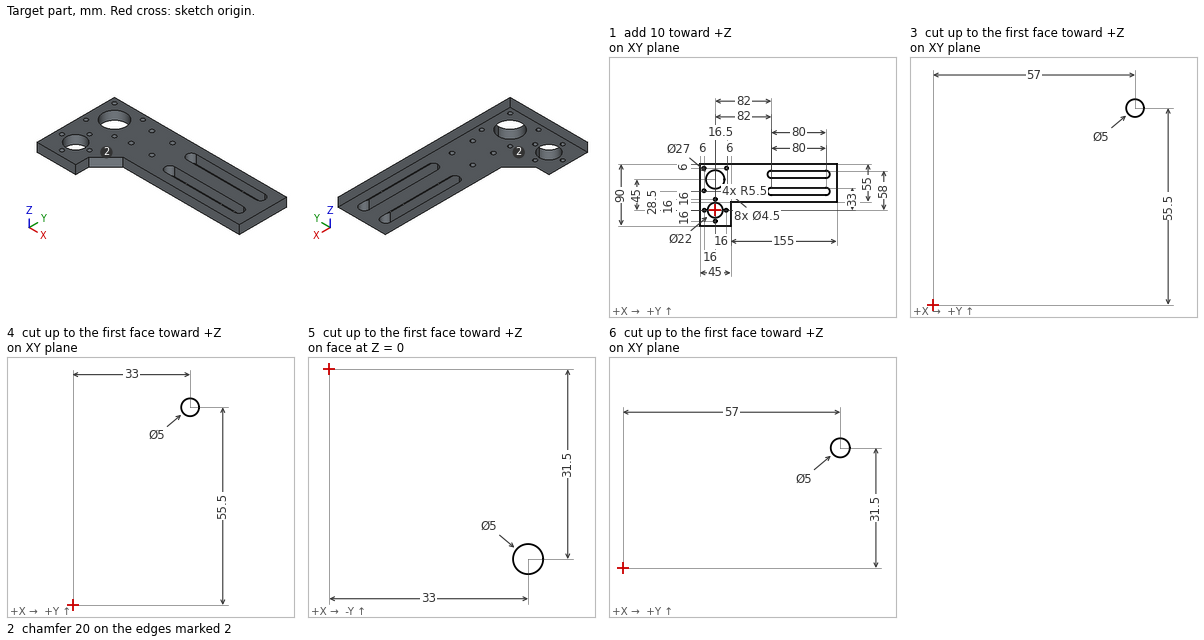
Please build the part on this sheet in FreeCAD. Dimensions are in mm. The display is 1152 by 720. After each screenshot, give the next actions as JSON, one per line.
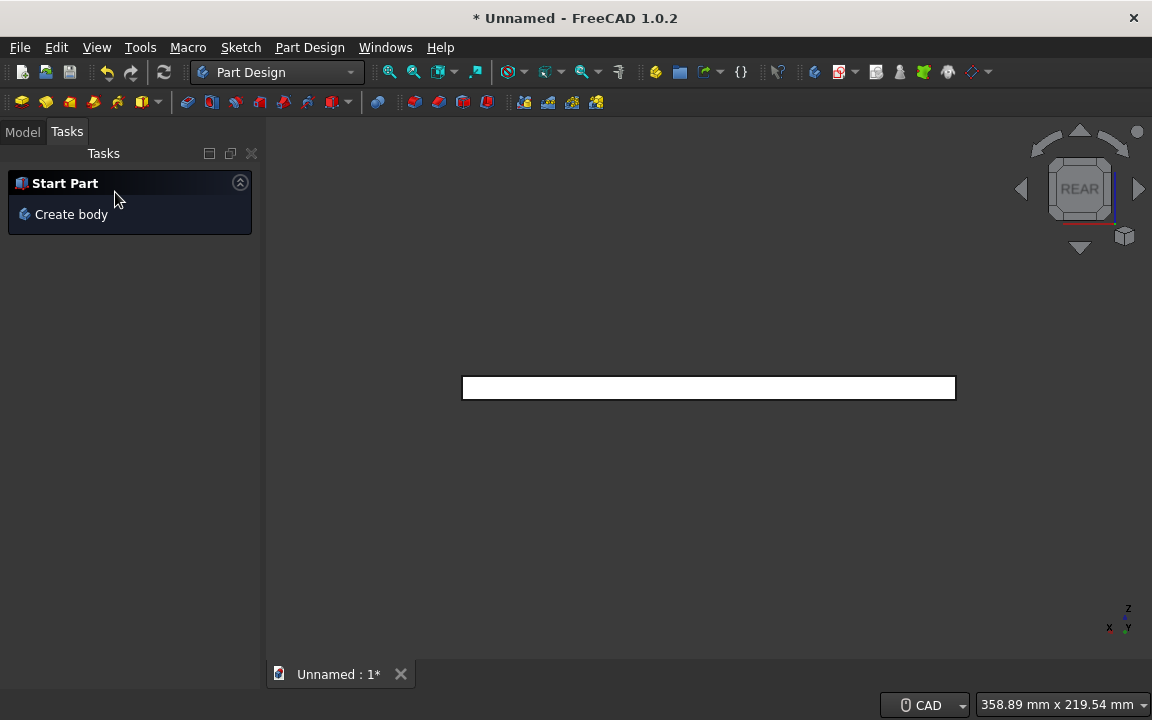
{"action": "key", "text": "6"}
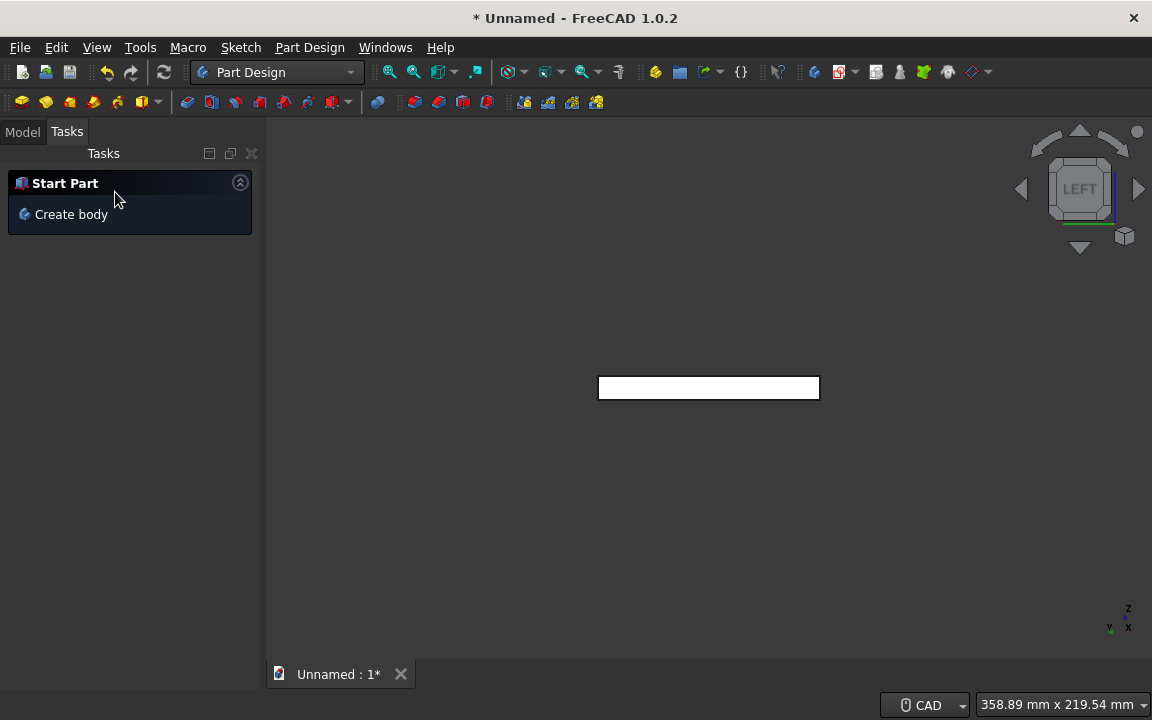
{"action": "key", "text": "v f"}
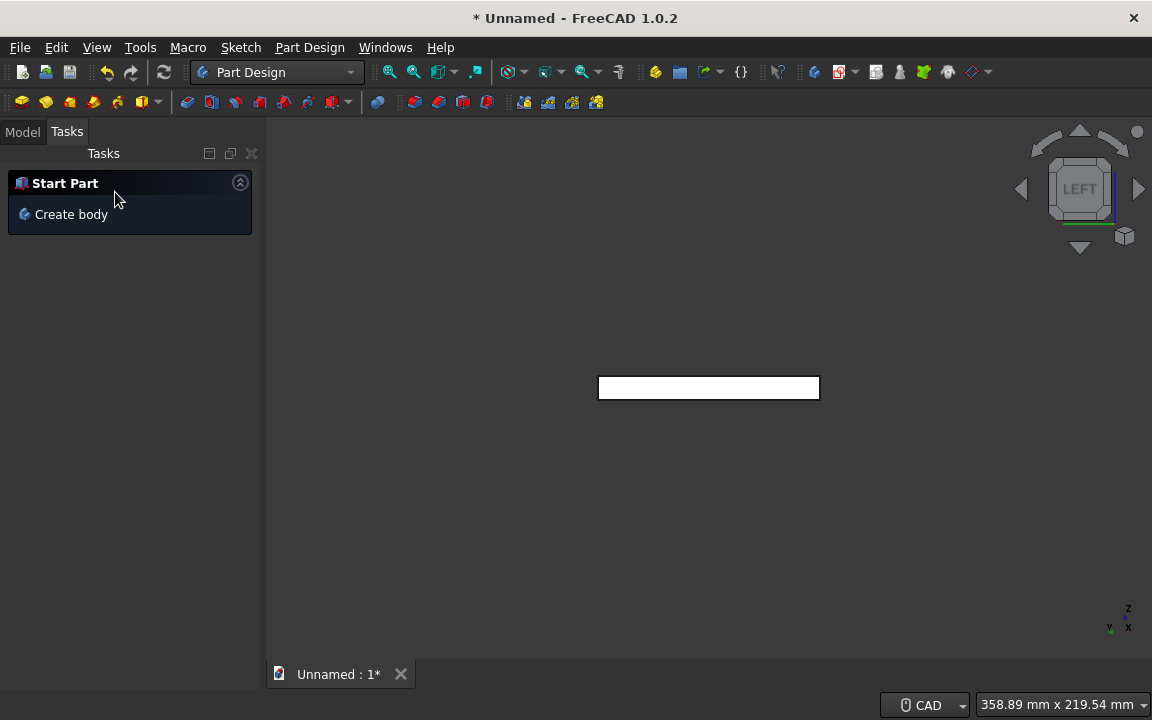
{"action": "key", "text": "v 3"}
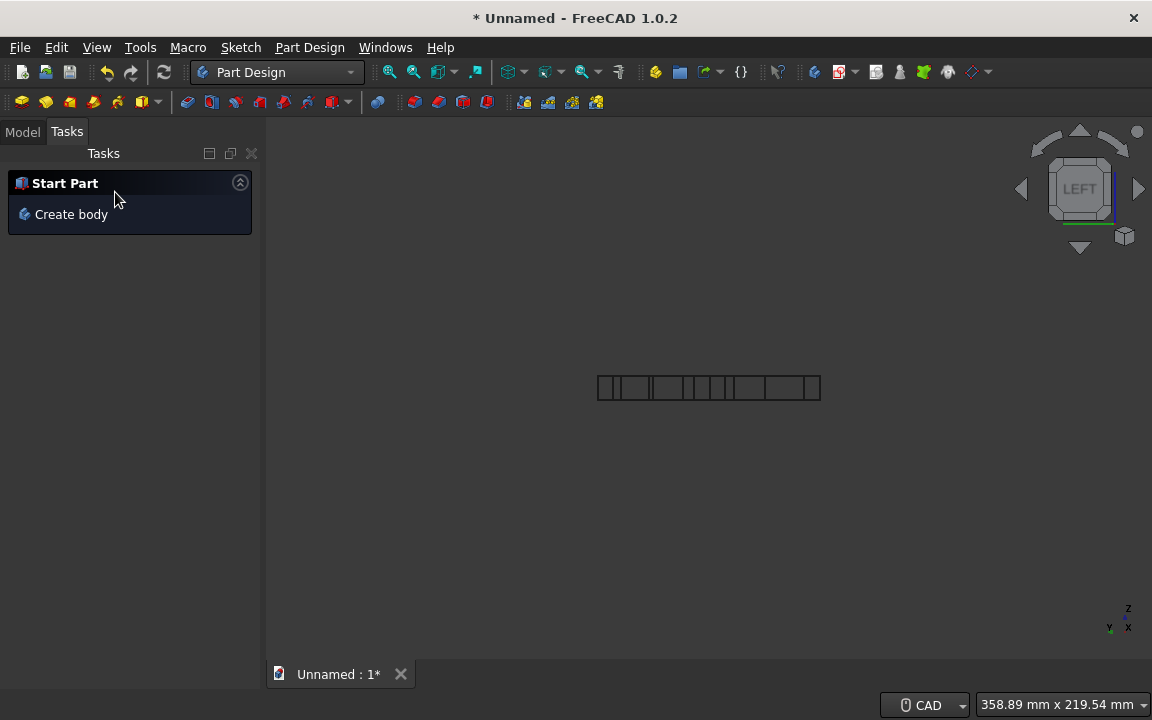
{"action": "key", "text": "0"}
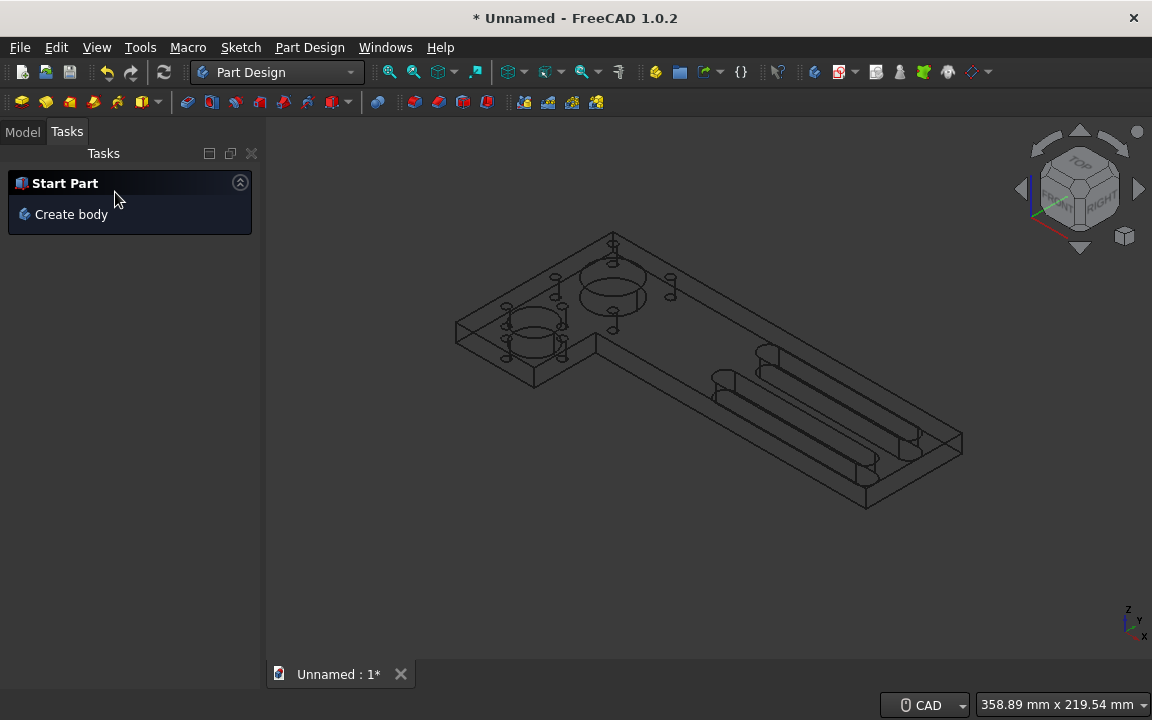
{"action": "left_click", "coordinate": [596, 342]}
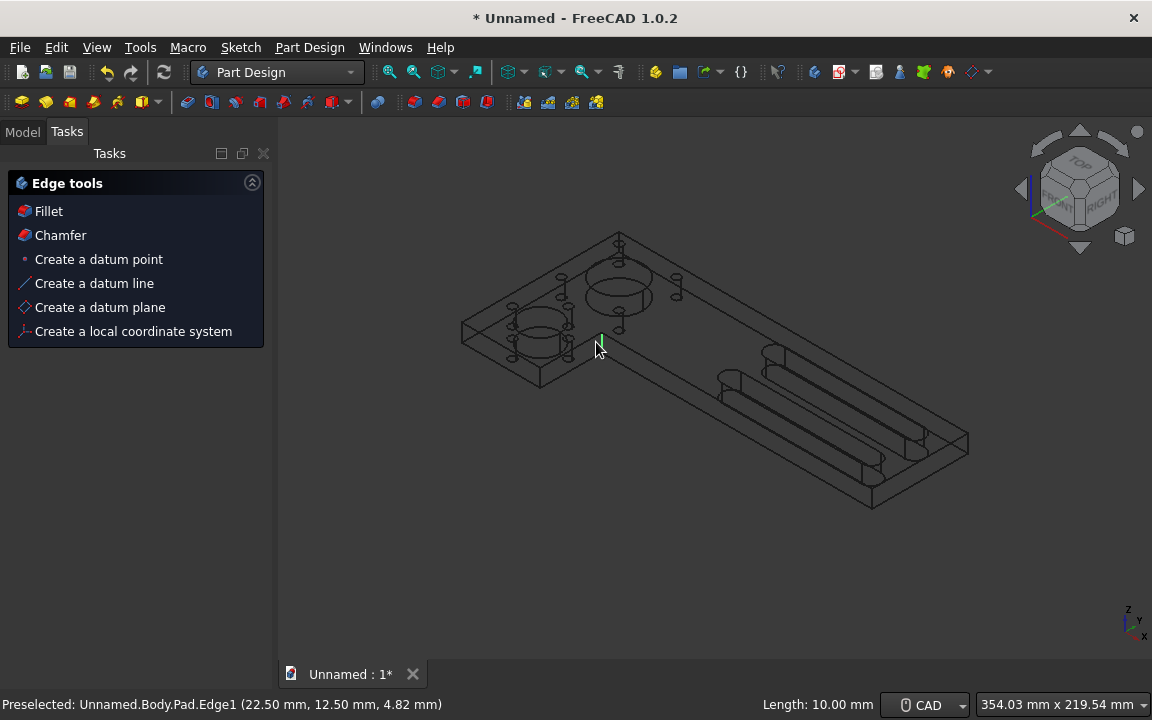
{"action": "key", "text": "v 1"}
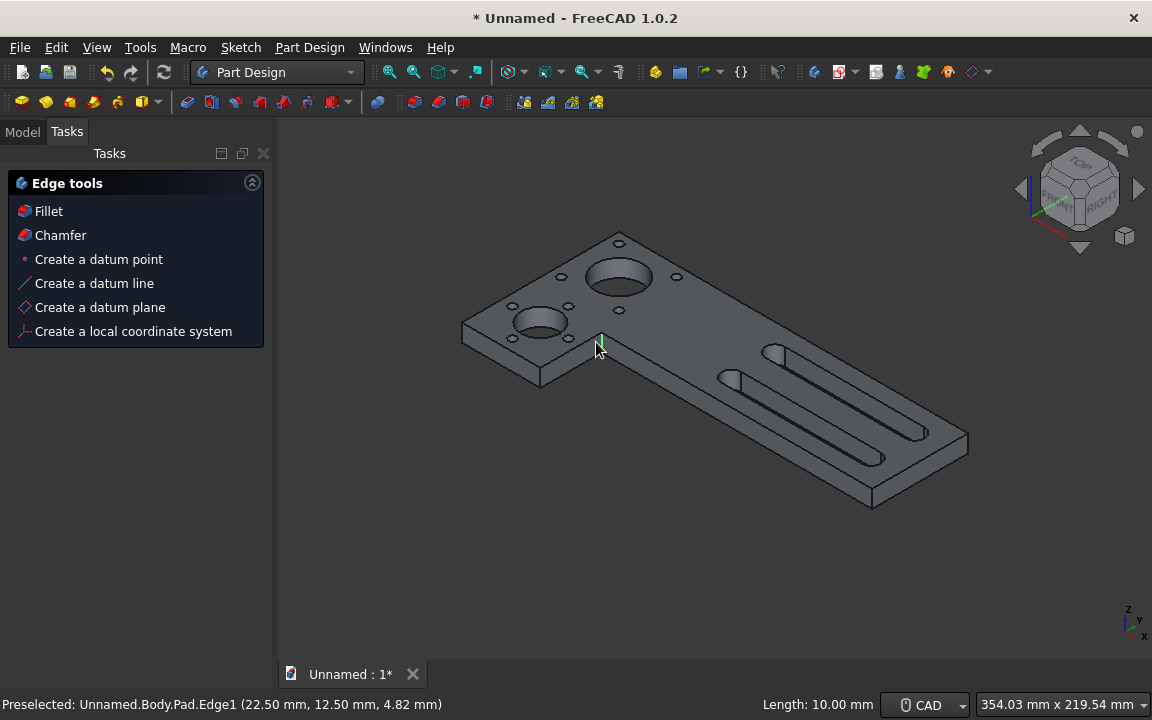
{"action": "left_click", "coordinate": [440, 102]}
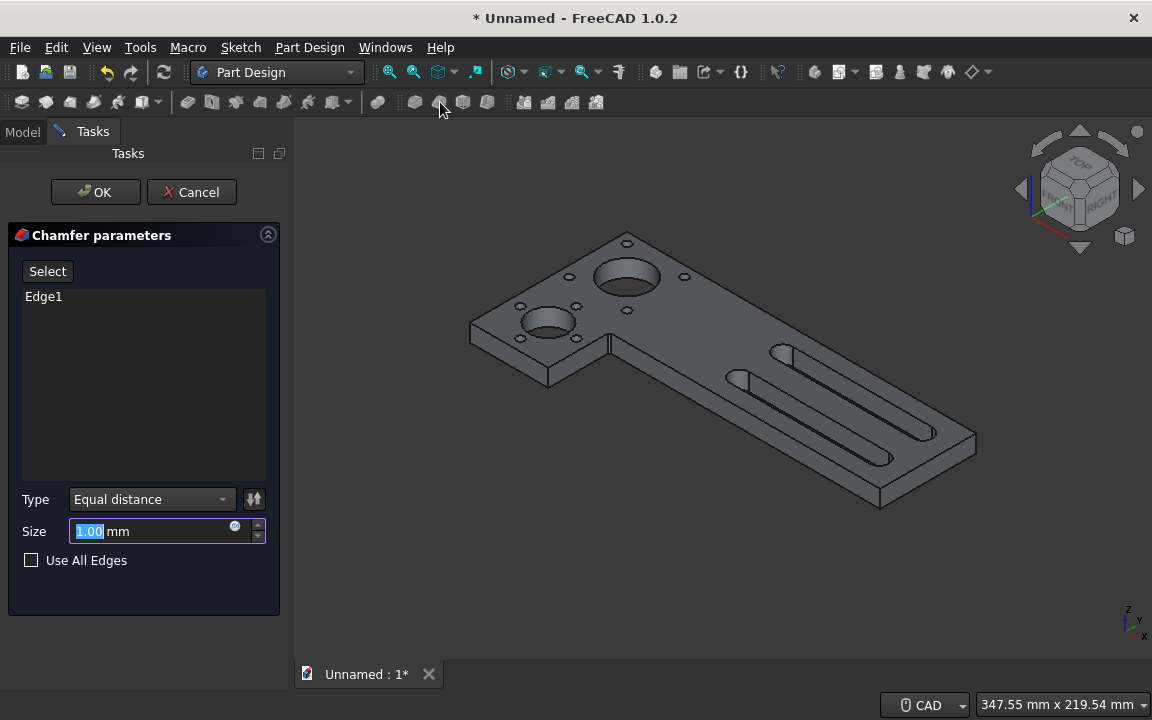
{"action": "type", "text": "20"}
{"action": "key", "text": "Tab"}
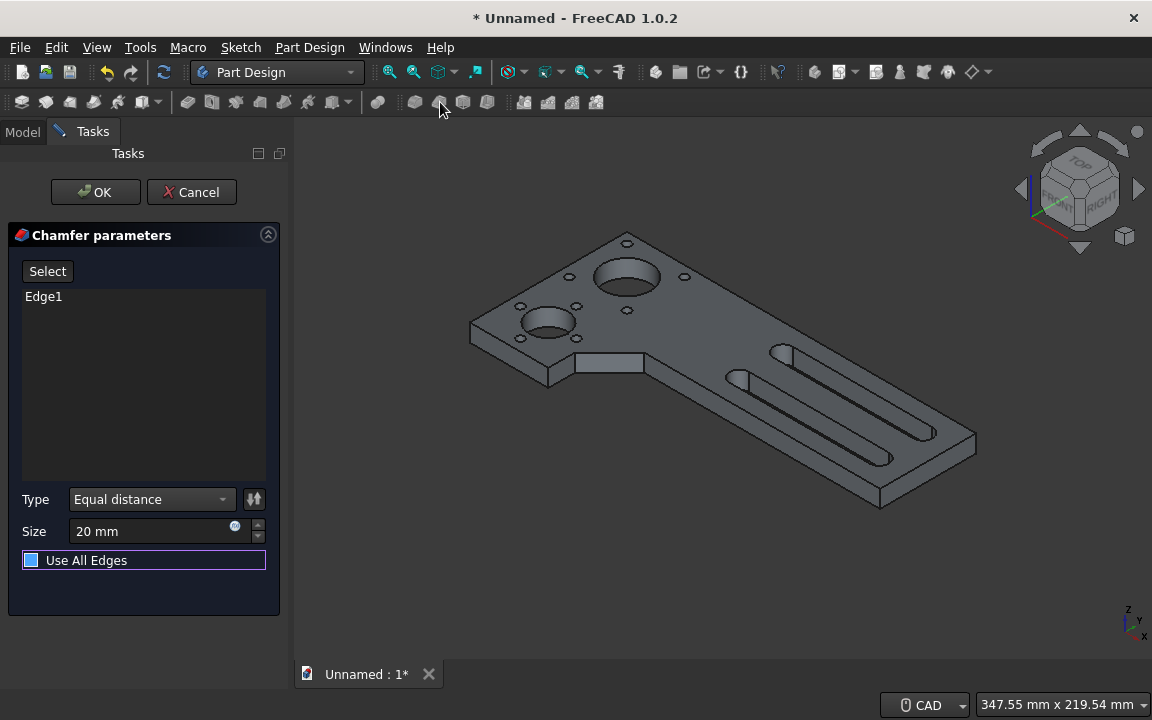
{"action": "left_click", "coordinate": [96, 192]}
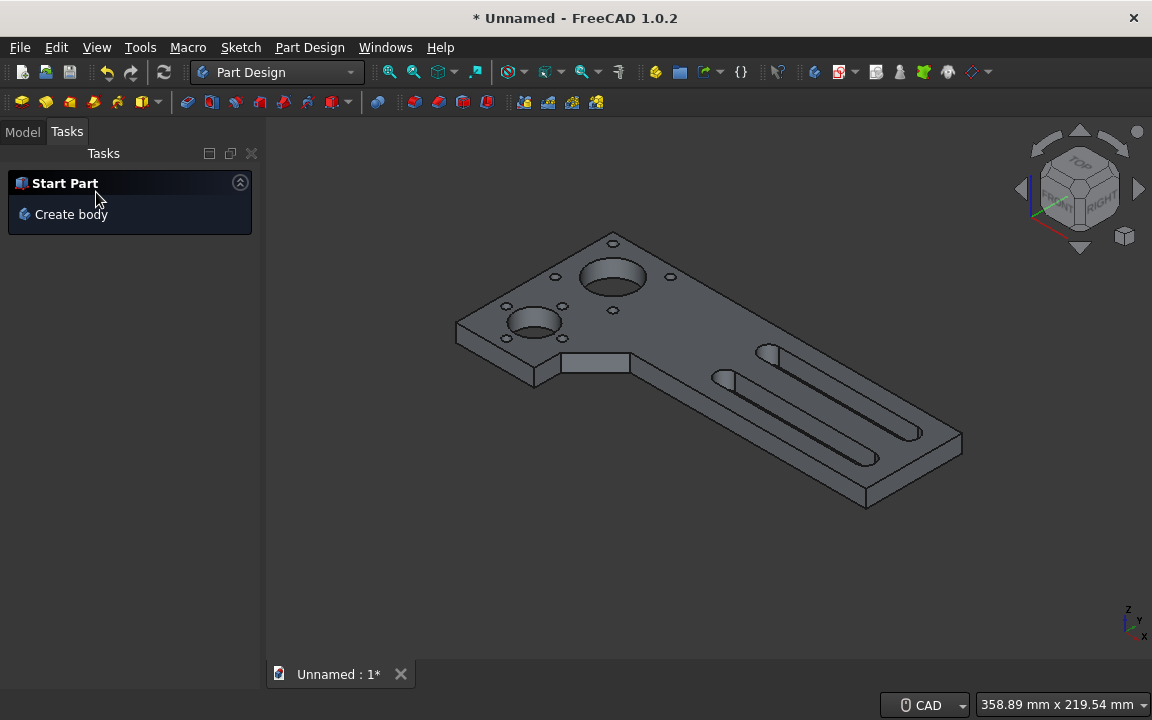
{"action": "left_click", "coordinate": [840, 72]}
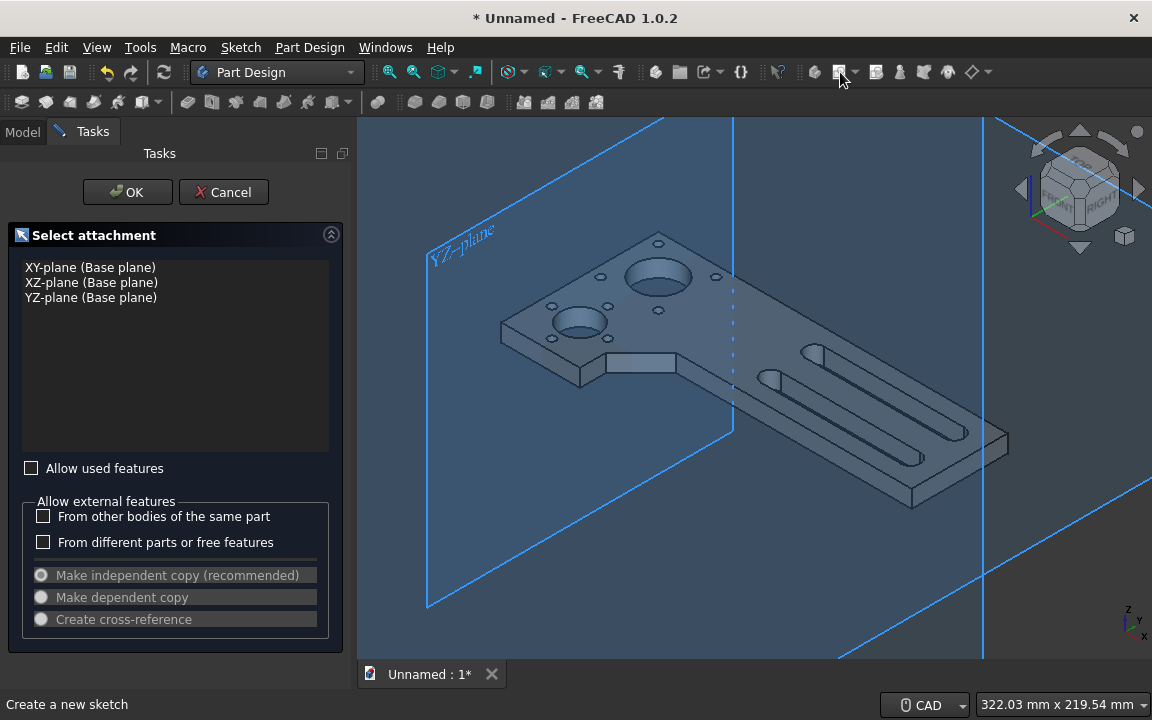
{"action": "left_click", "coordinate": [82, 268]}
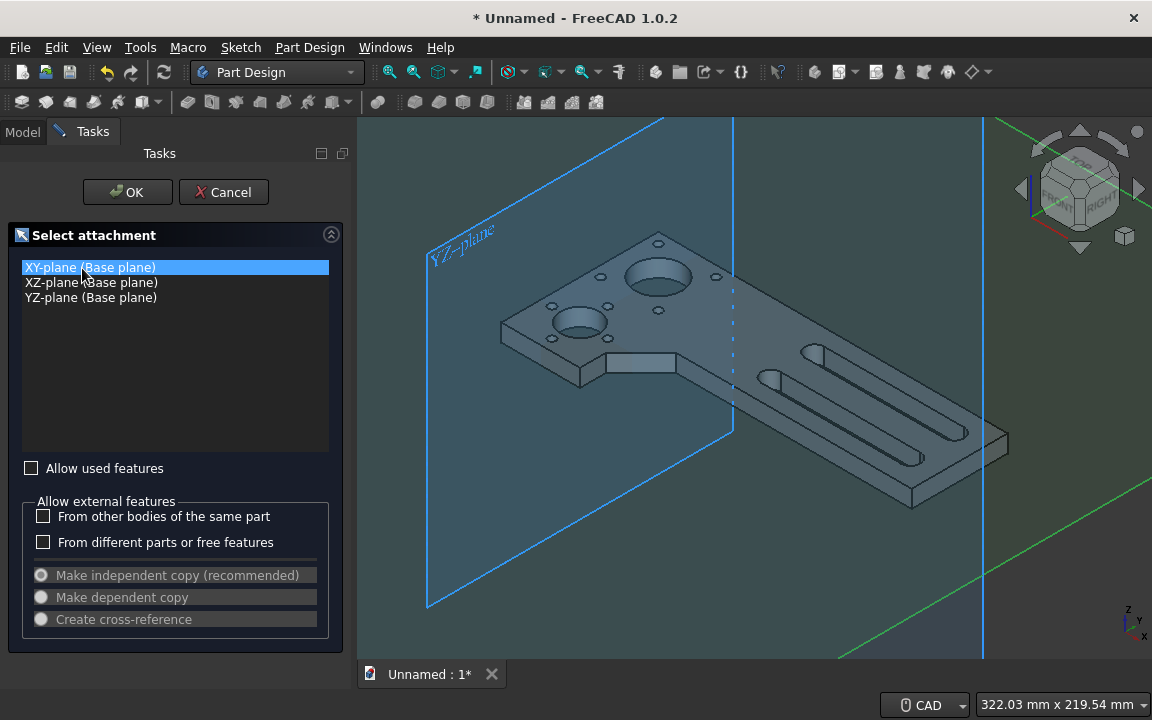
{"action": "left_click", "coordinate": [128, 192]}